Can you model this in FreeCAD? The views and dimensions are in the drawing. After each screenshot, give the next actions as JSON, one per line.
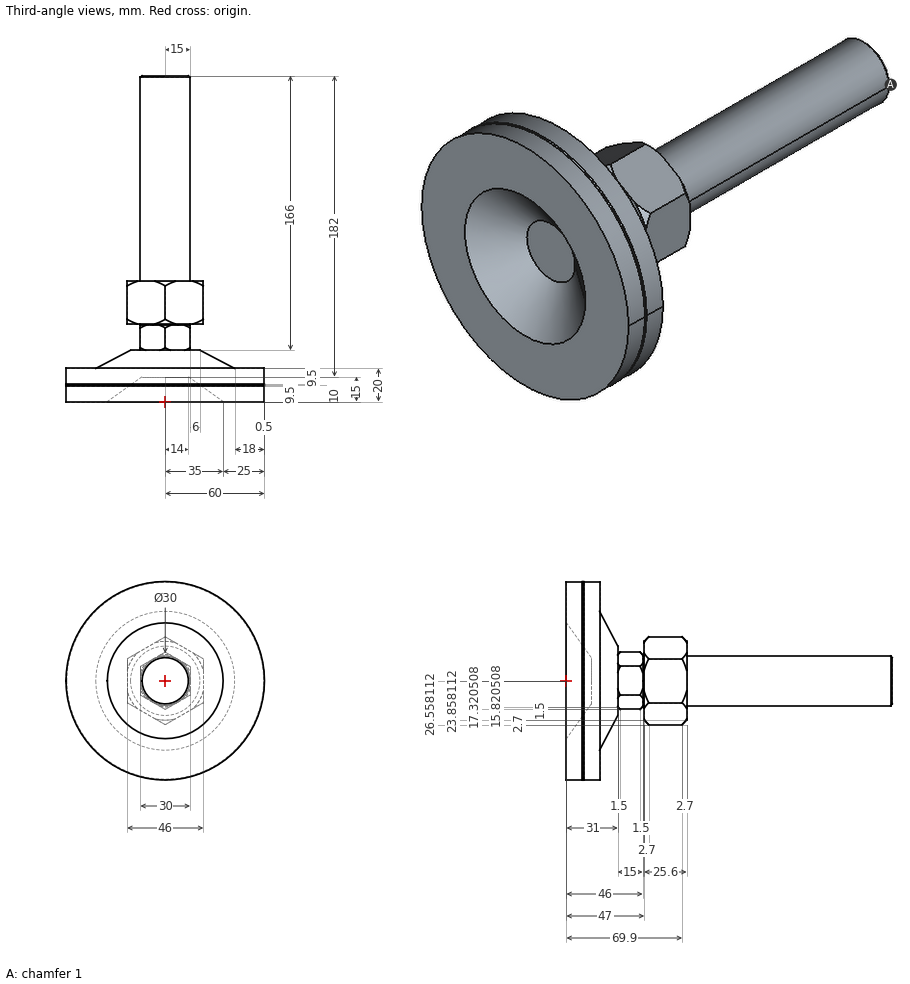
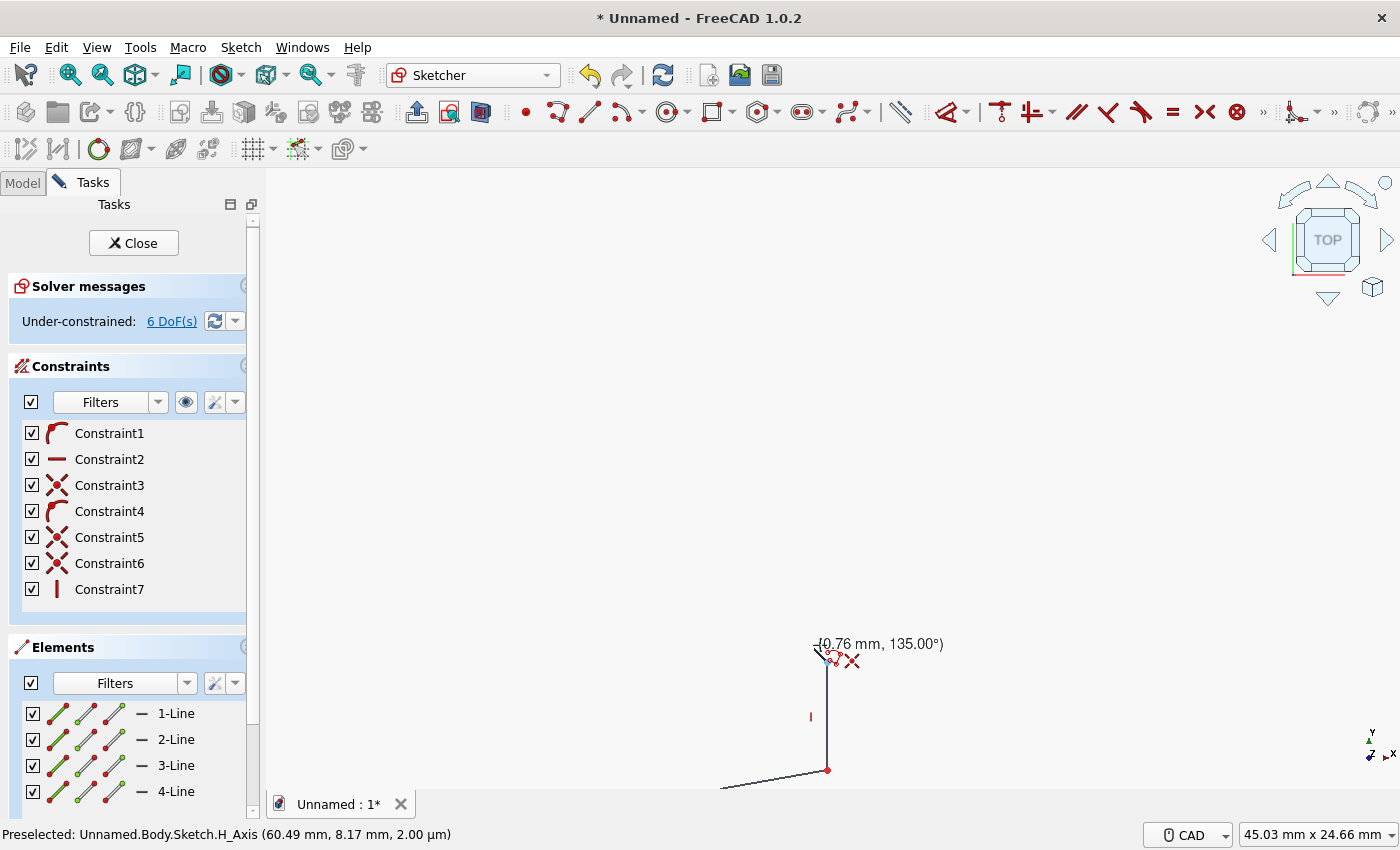
{"action": "left_click", "coordinate": [816, 630]}
{"action": "left_click", "coordinate": [828, 617]}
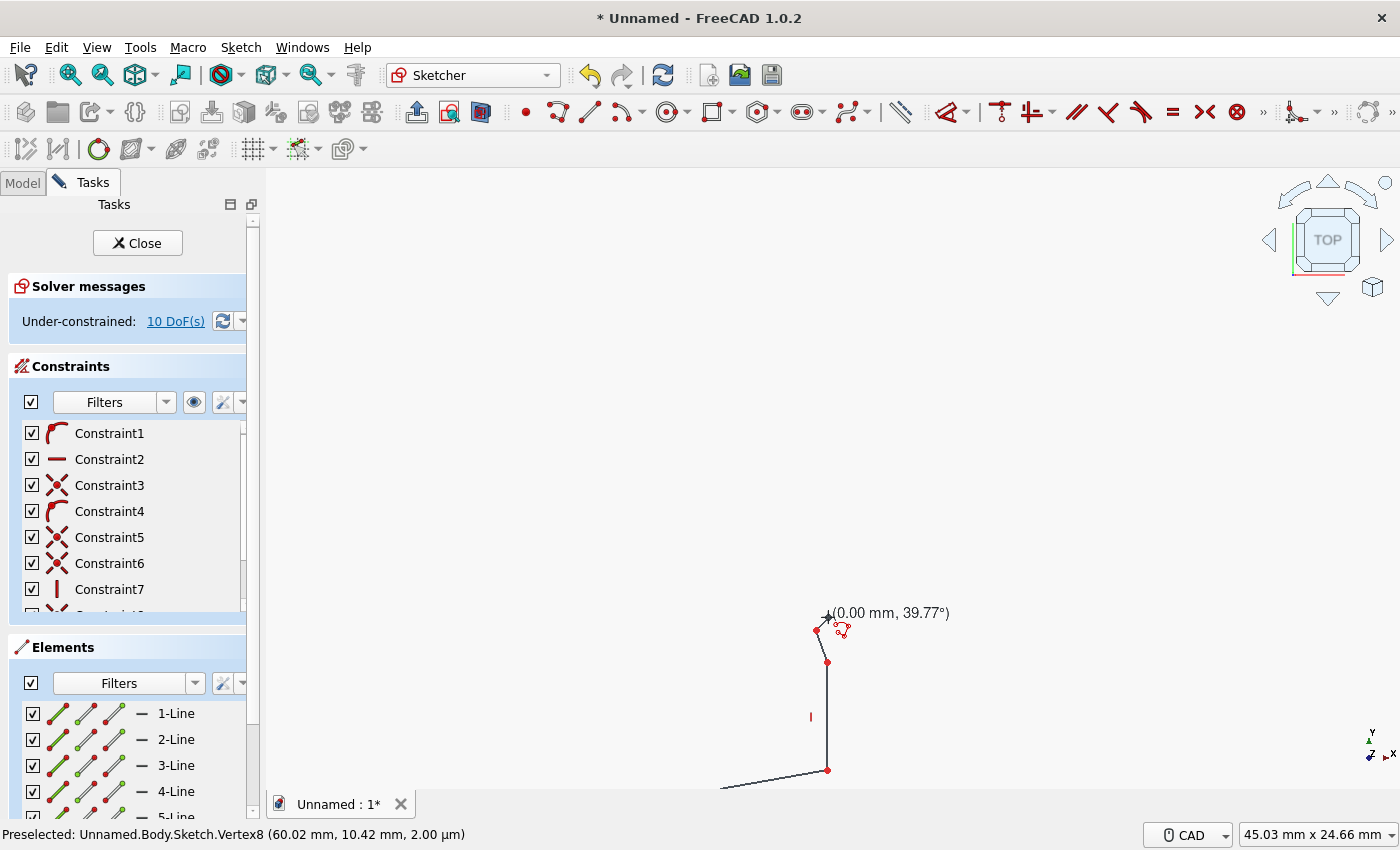
{"action": "scroll", "coordinate": [820, 645], "scroll_direction": "down", "scroll_amount": 13}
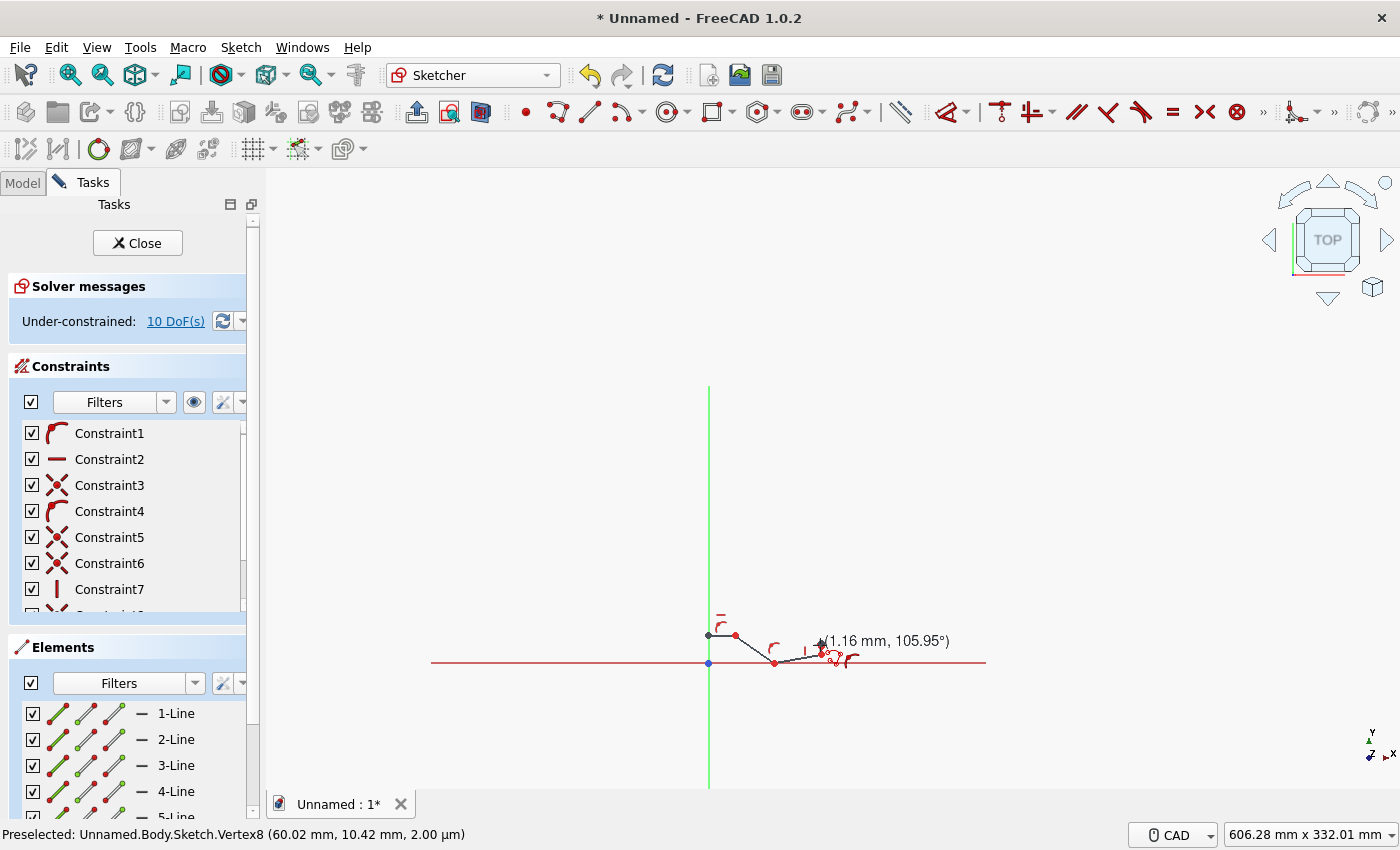
{"action": "left_click", "coordinate": [821, 626]}
{"action": "left_click", "coordinate": [787, 626]}
{"action": "left_click", "coordinate": [748, 605]}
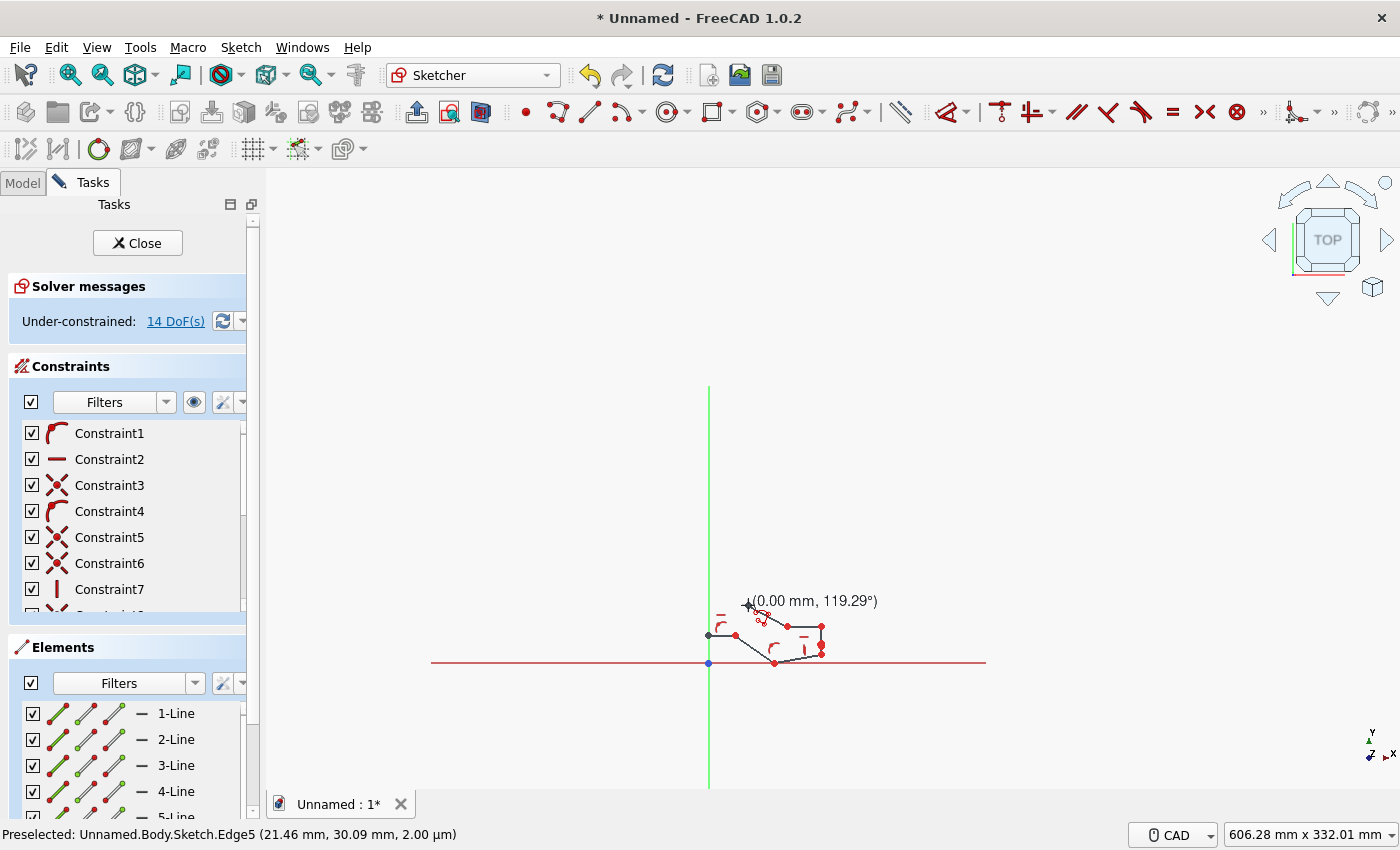
{"action": "scroll", "coordinate": [737, 605], "scroll_direction": "up", "scroll_amount": 2}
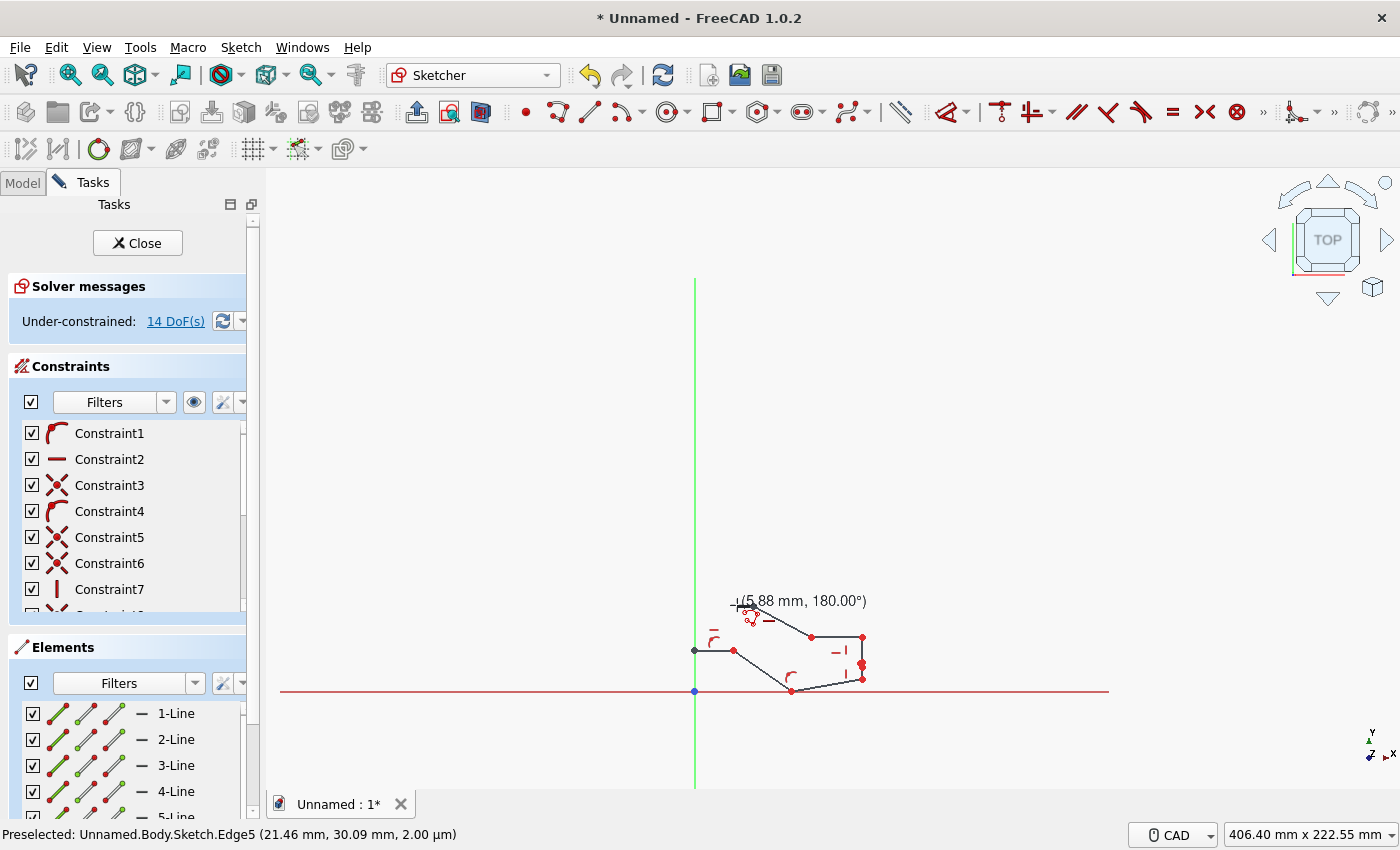
{"action": "left_click", "coordinate": [737, 605]}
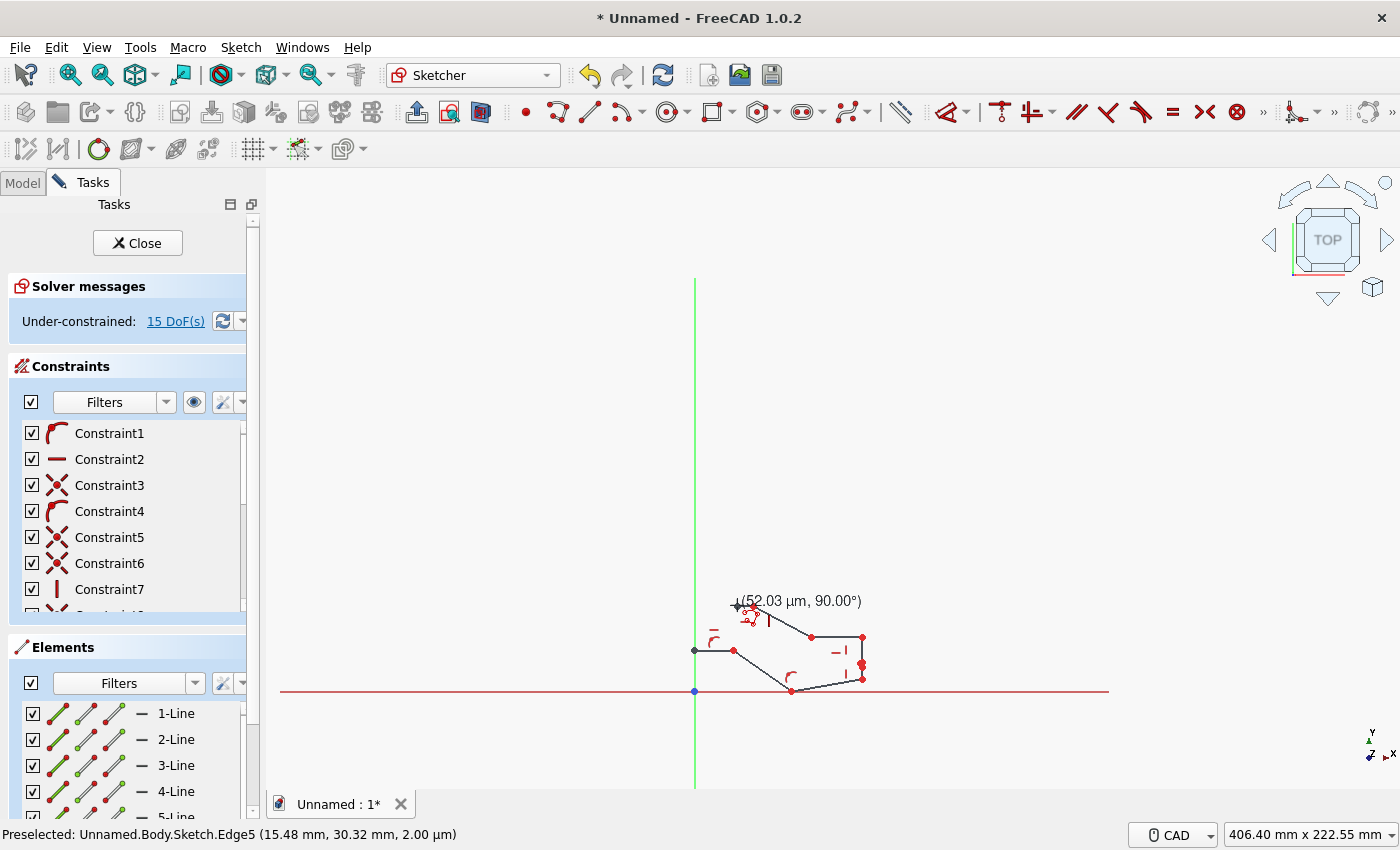
{"action": "scroll", "coordinate": [736, 604], "scroll_direction": "down", "scroll_amount": 2}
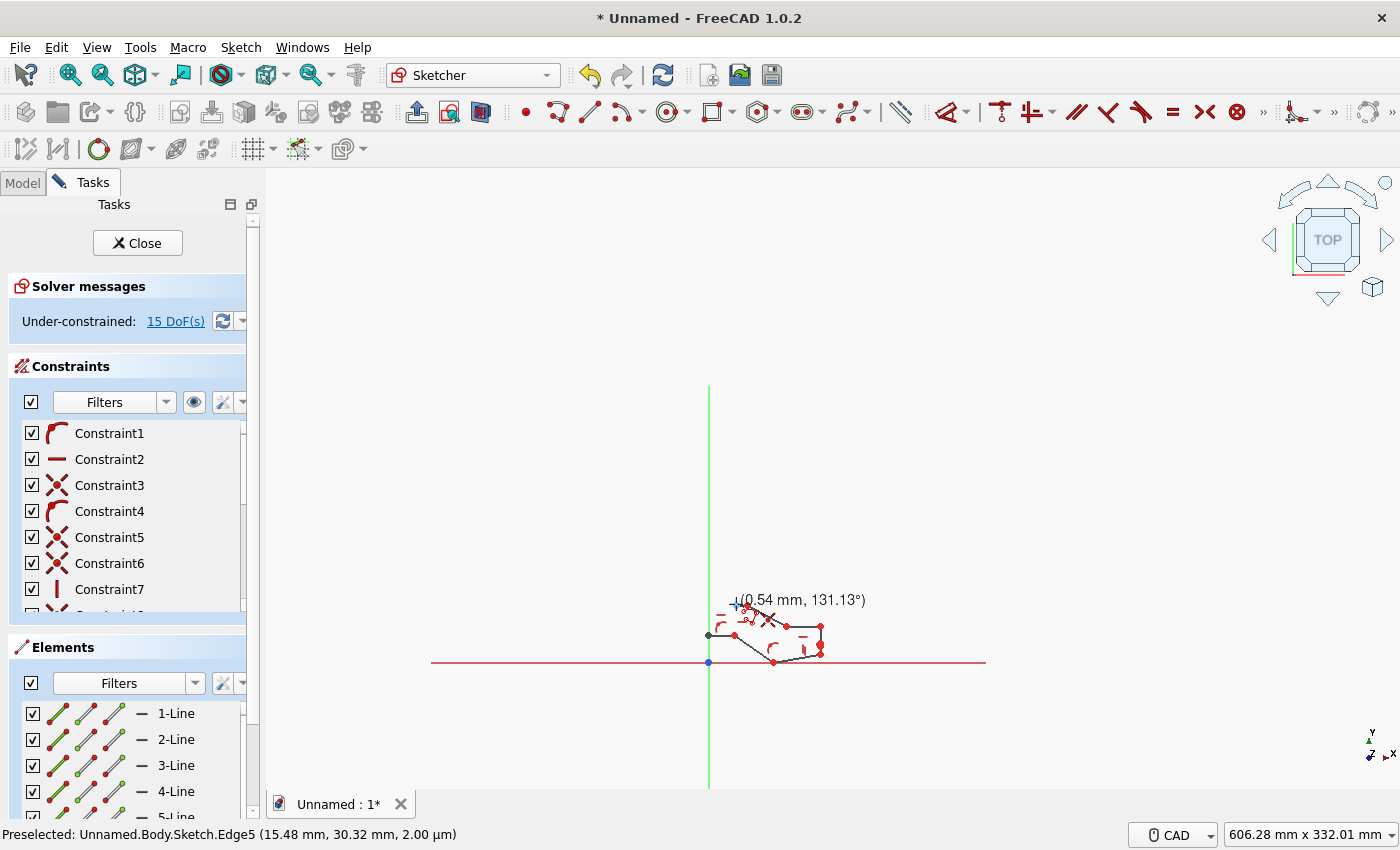
{"action": "left_click", "coordinate": [737, 294]}
{"action": "left_click", "coordinate": [718, 294]}
{"action": "left_click", "coordinate": [709, 636]}
{"action": "key", "text": "Escape"}
{"action": "key", "text": "Escape"}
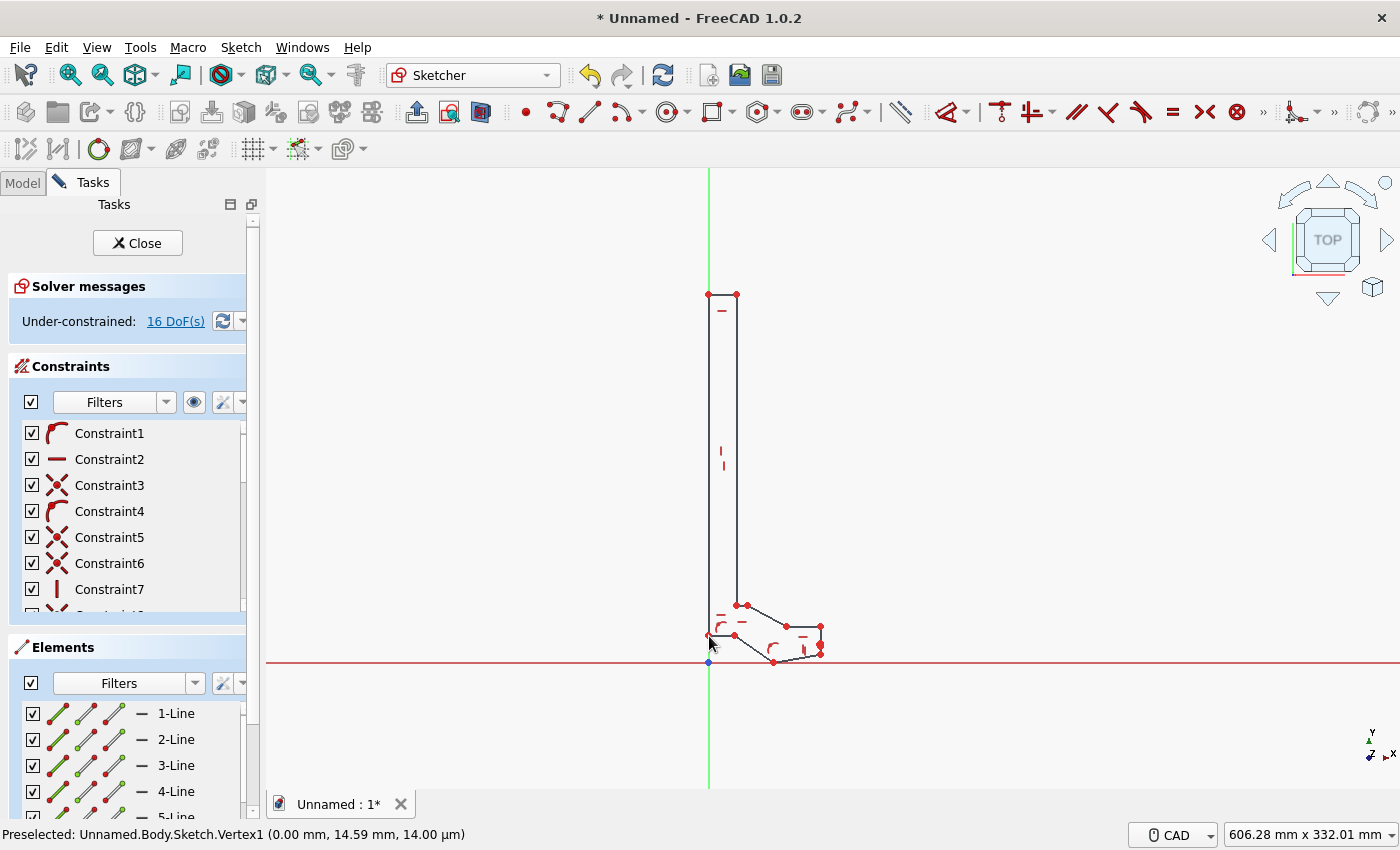
{"action": "left_click", "coordinate": [788, 660]}